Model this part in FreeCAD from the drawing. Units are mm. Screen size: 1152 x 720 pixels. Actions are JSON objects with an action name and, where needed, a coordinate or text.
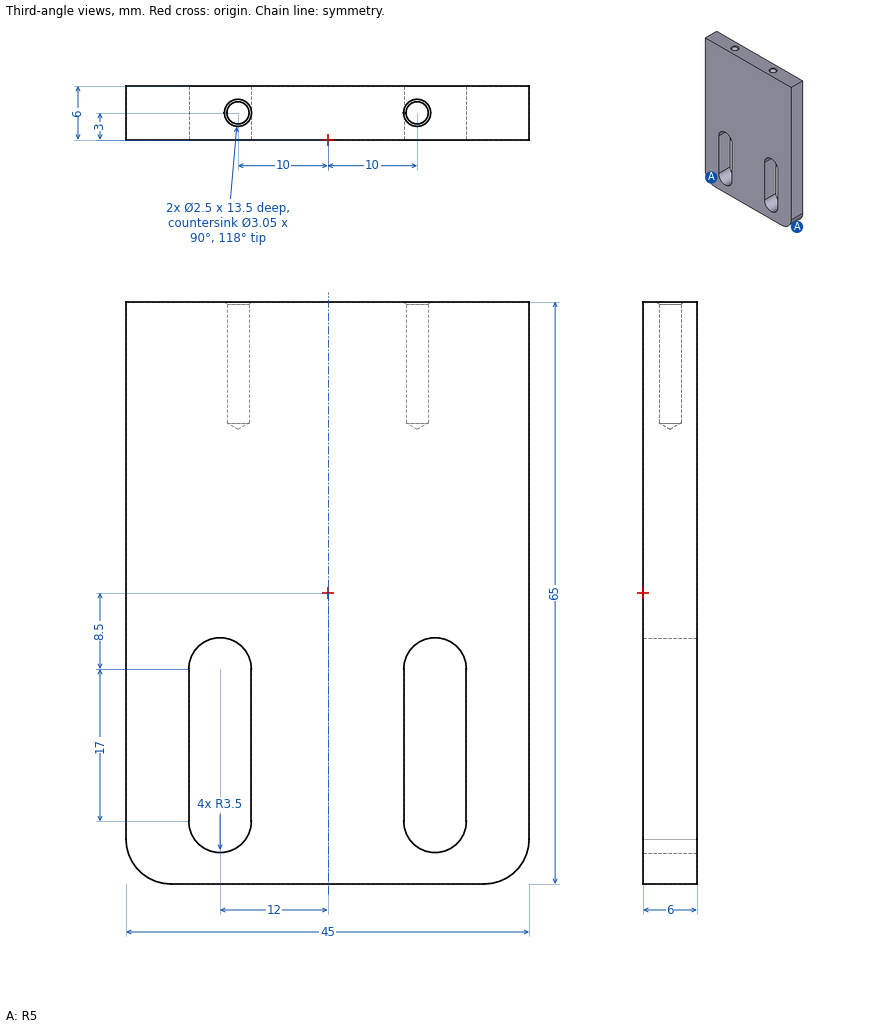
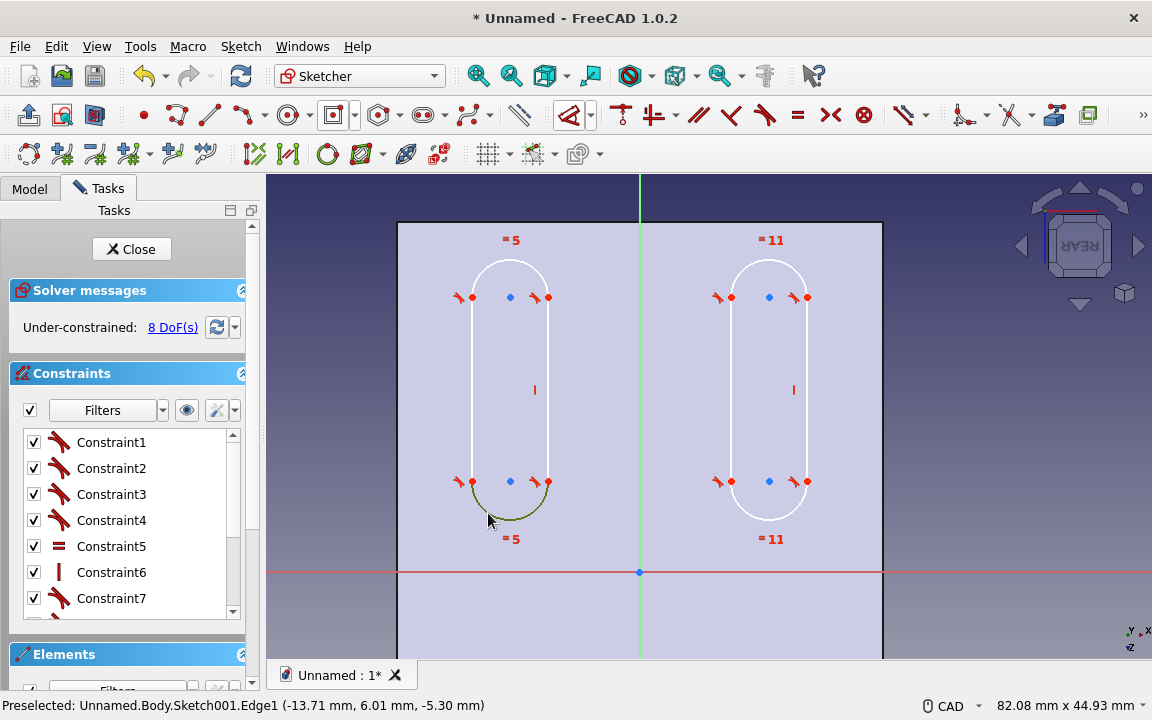
{"action": "left_click", "coordinate": [747, 513]}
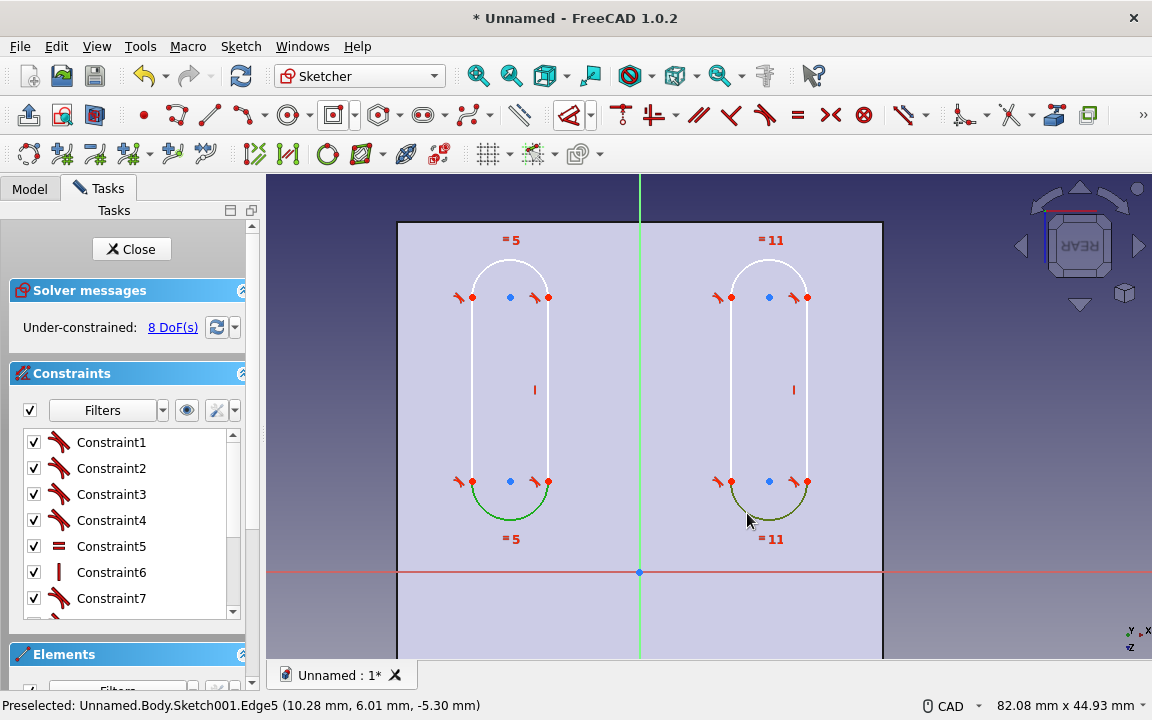
{"action": "key", "text": "e"}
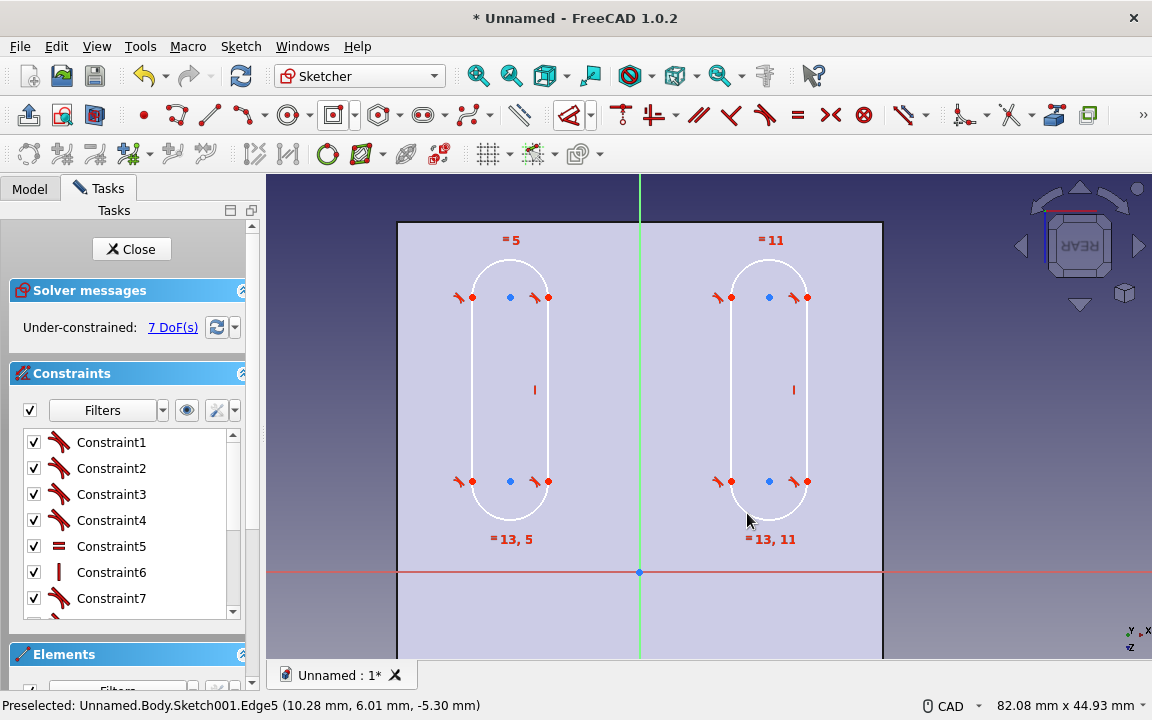
{"action": "left_click", "coordinate": [510, 482]}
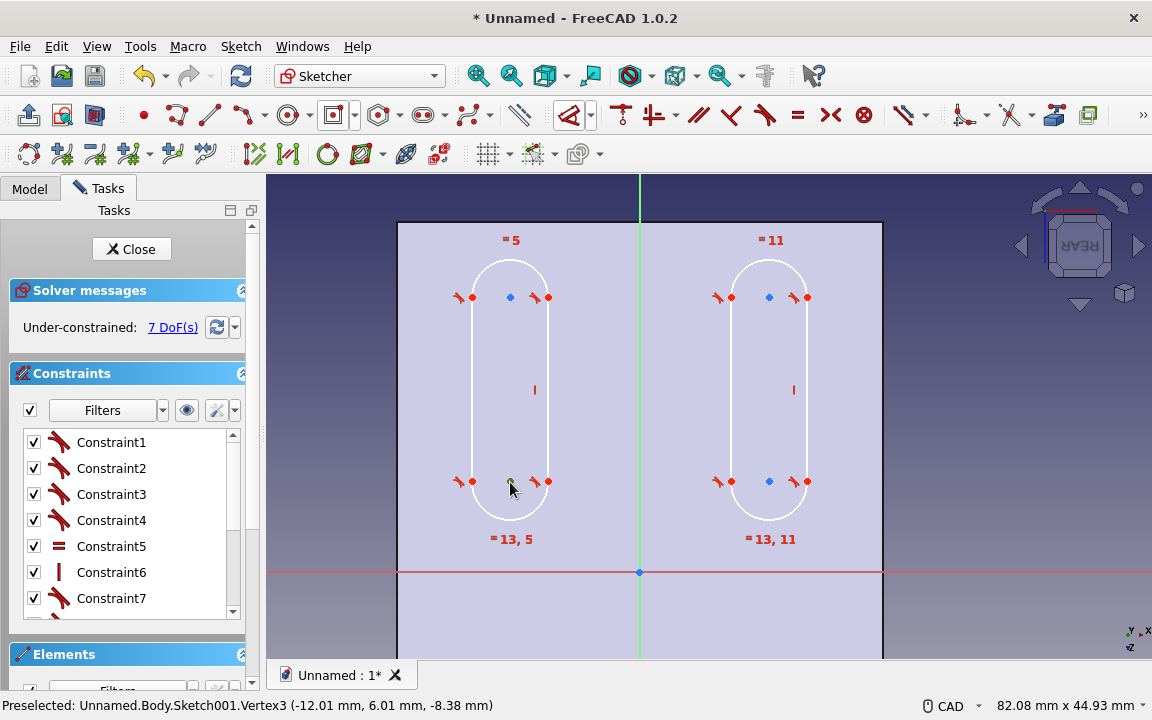
{"action": "left_click", "coordinate": [769, 482]}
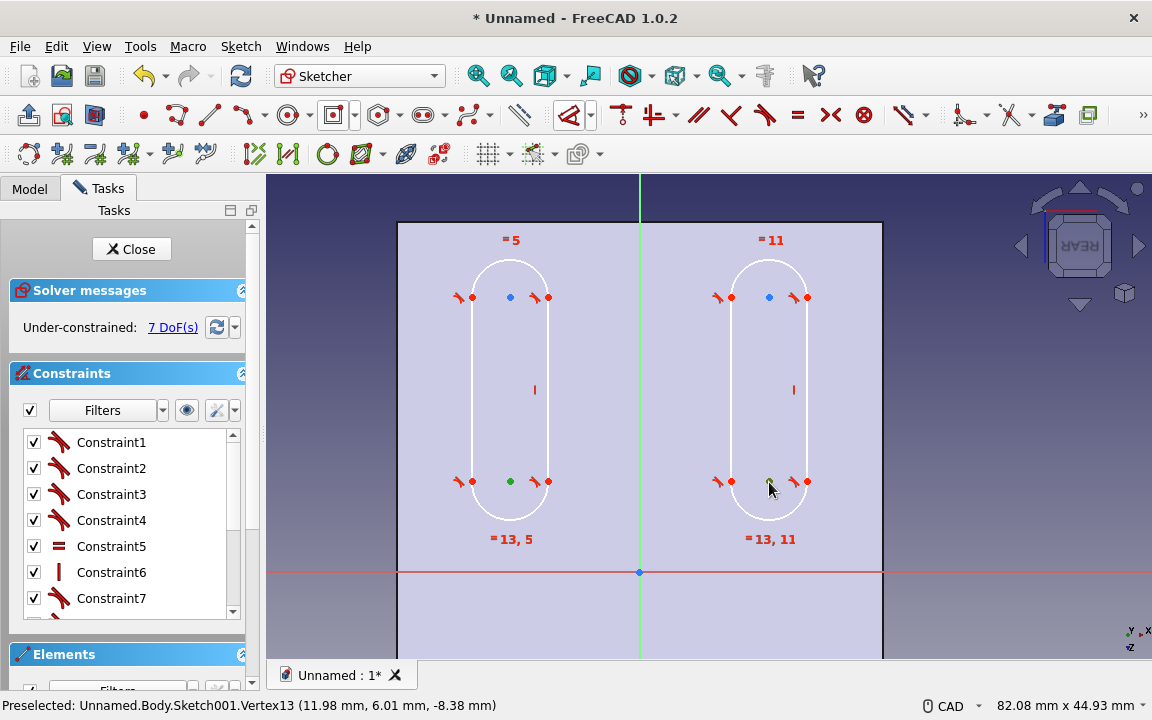
{"action": "left_click", "coordinate": [640, 539]}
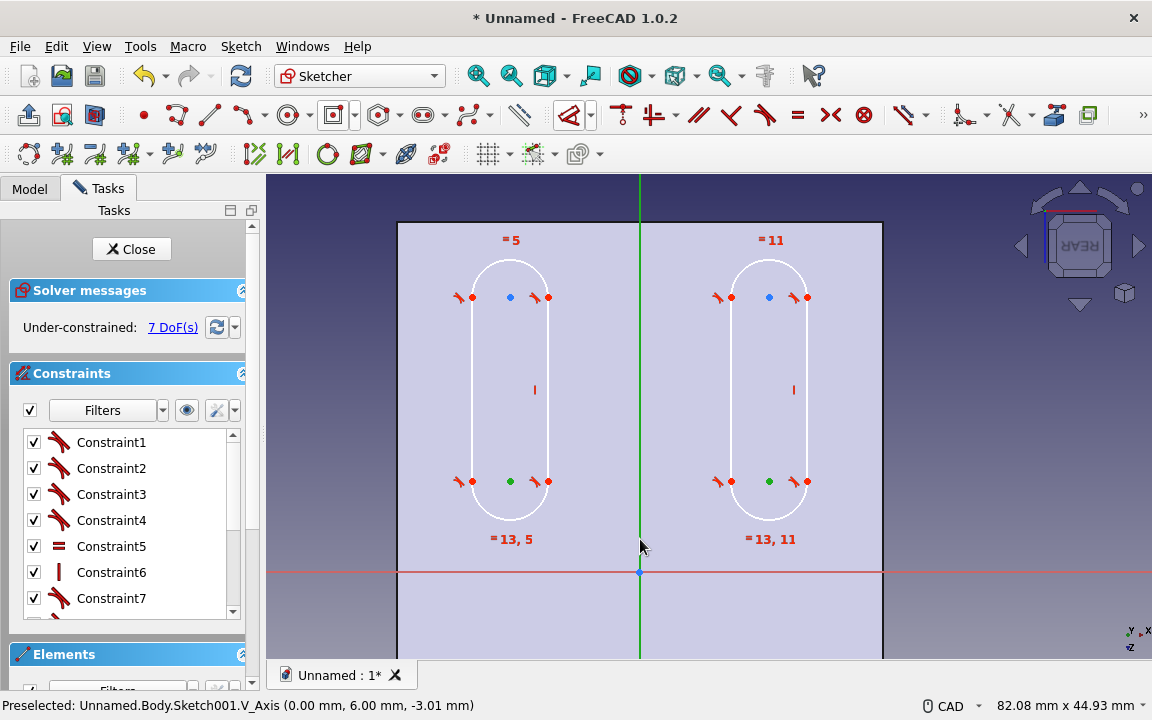
{"action": "key", "text": "s"}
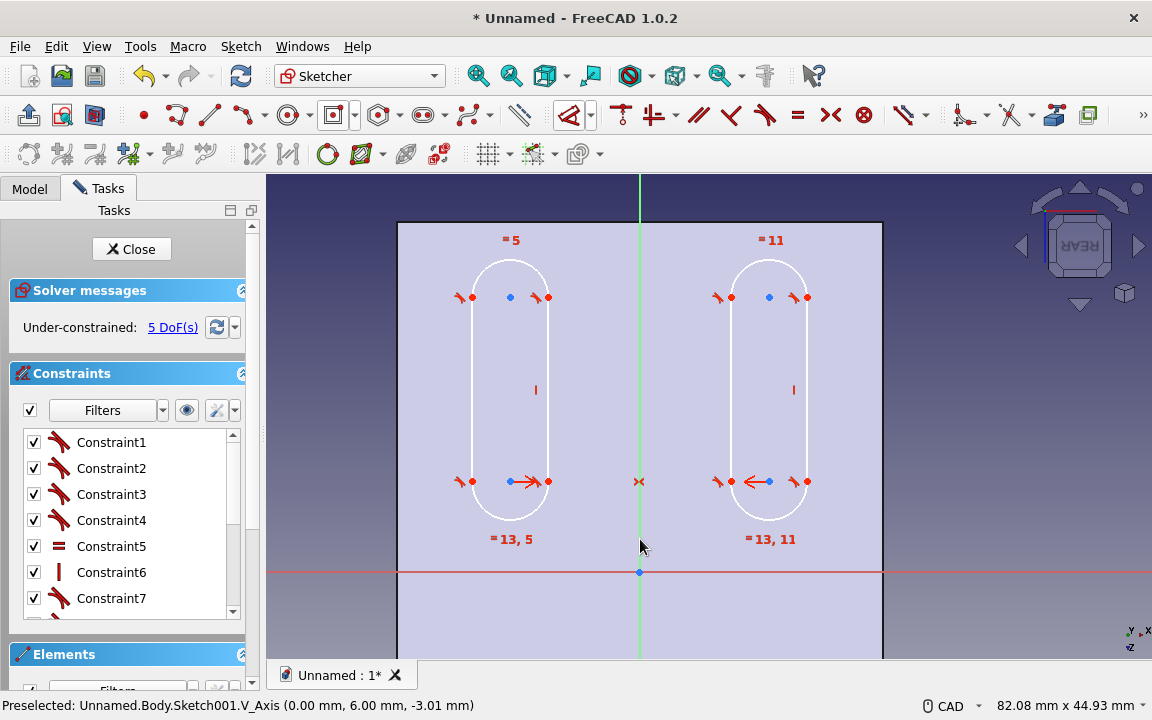
{"action": "key", "text": "d"}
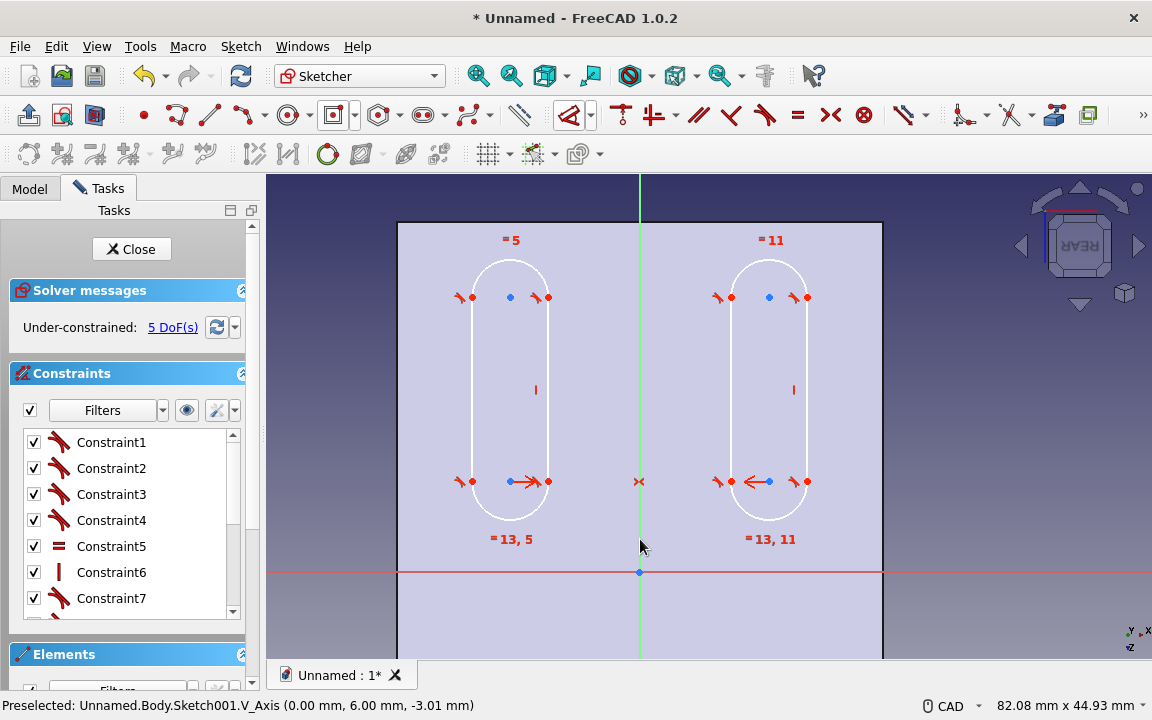
{"action": "left_click", "coordinate": [488, 513]}
{"action": "left_click", "coordinate": [469, 539]}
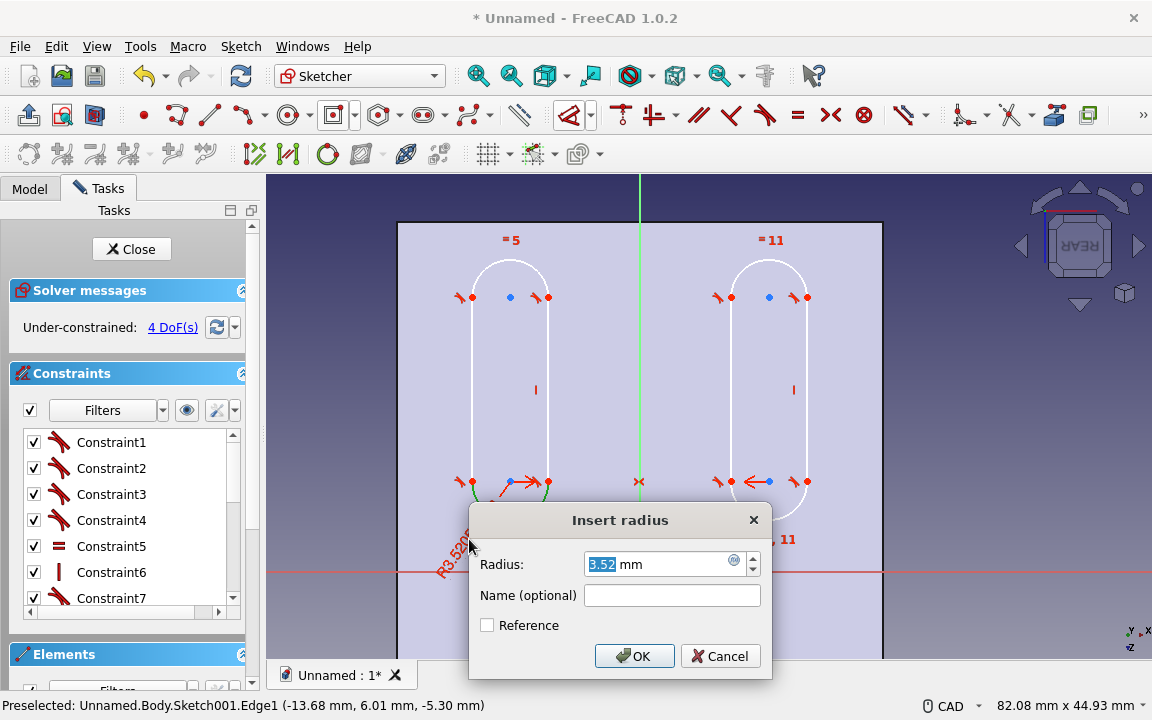
{"action": "type", "text": "3.5"}
{"action": "key", "text": "Return"}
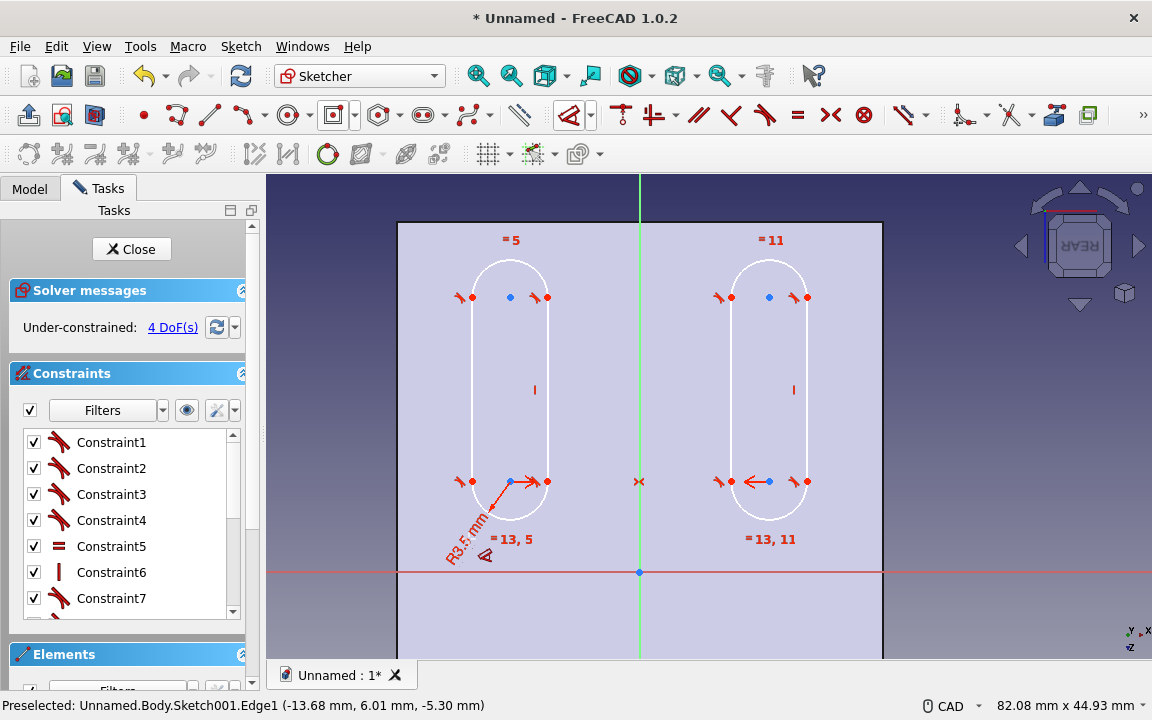
{"action": "left_click", "coordinate": [472, 427]}
{"action": "left_click", "coordinate": [438, 390]}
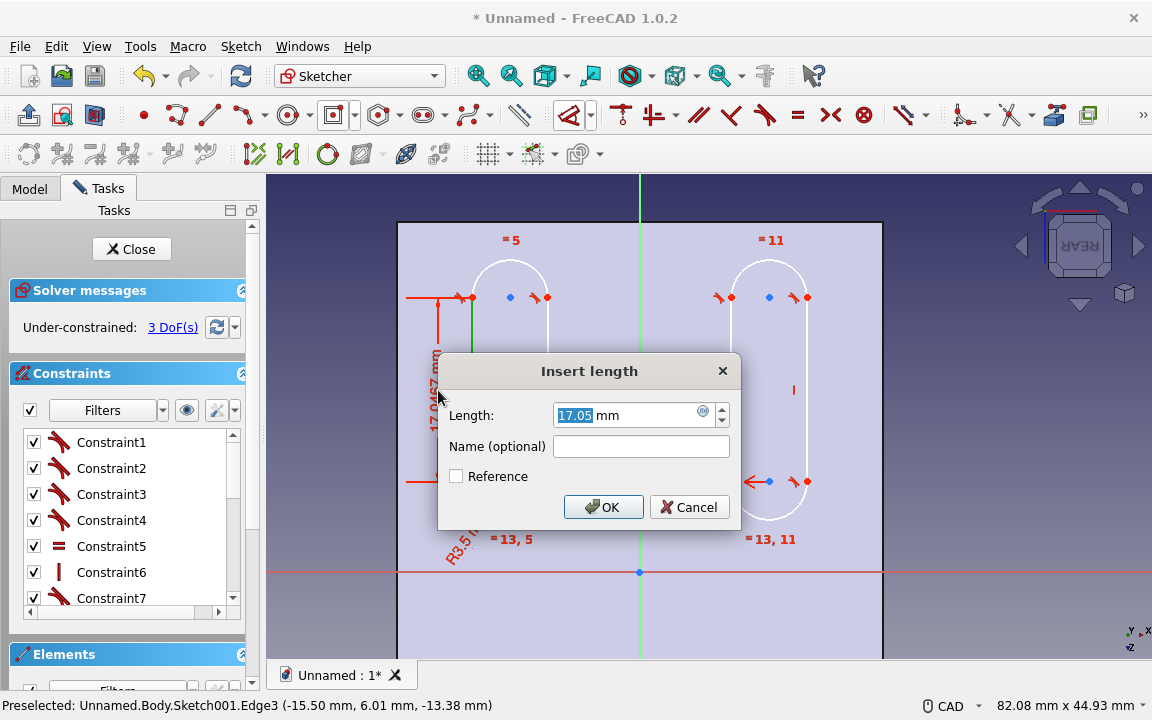
{"action": "type", "text": "17"}
{"action": "key", "text": "Return"}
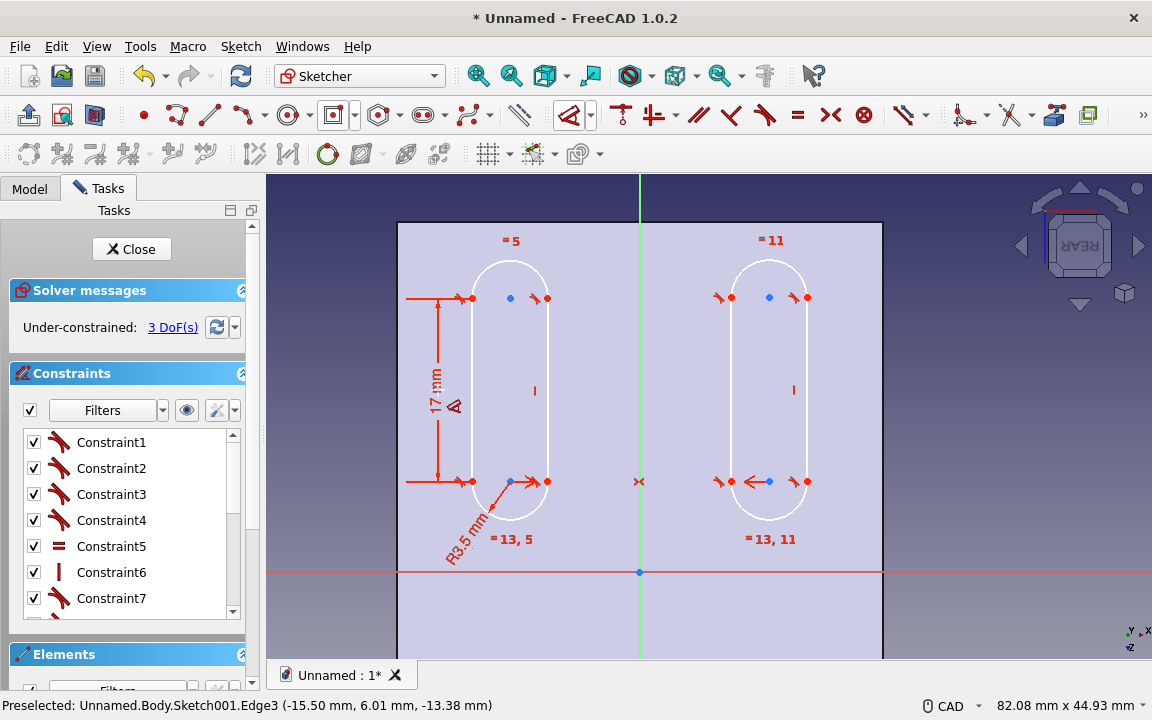
{"action": "left_click", "coordinate": [731, 427]}
{"action": "left_click", "coordinate": [765, 390]}